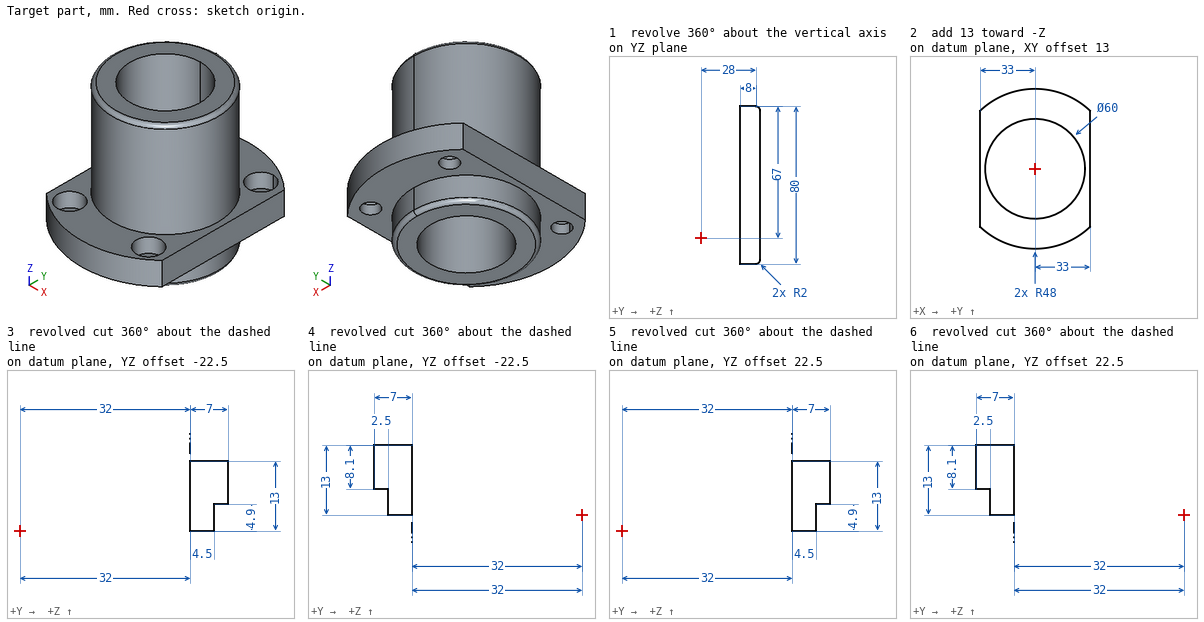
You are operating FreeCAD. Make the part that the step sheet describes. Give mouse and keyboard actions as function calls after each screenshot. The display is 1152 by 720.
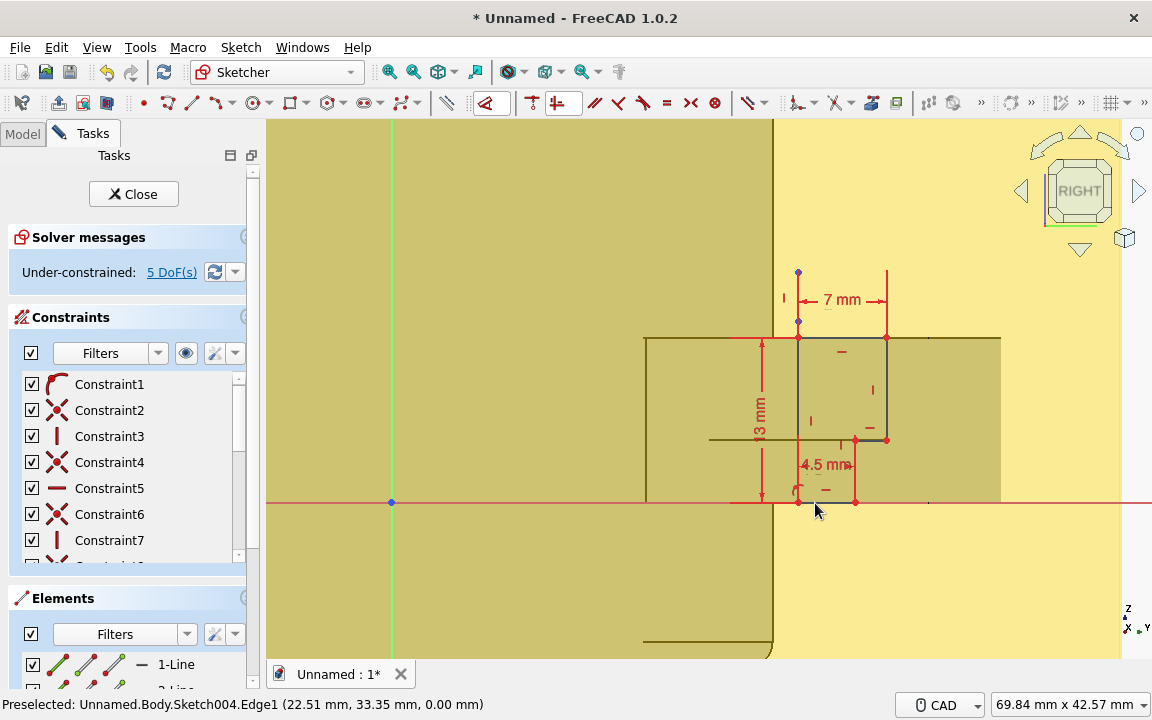
click(855, 484)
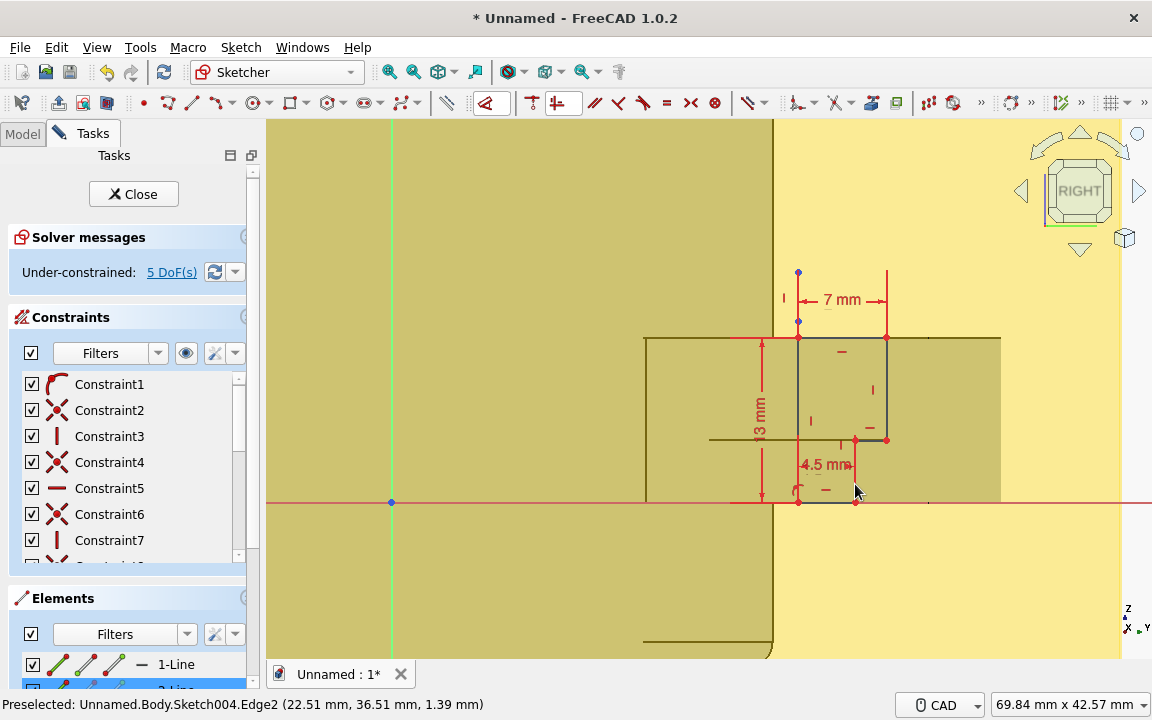
key(i)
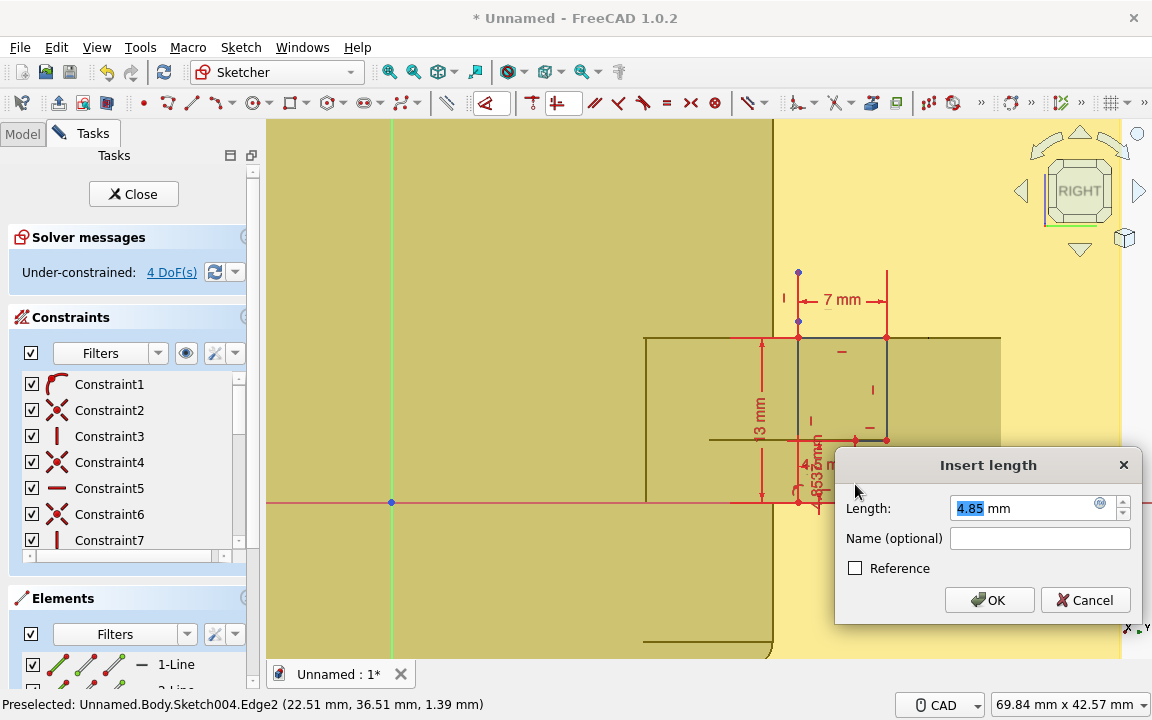
text(4.9)
key(Return)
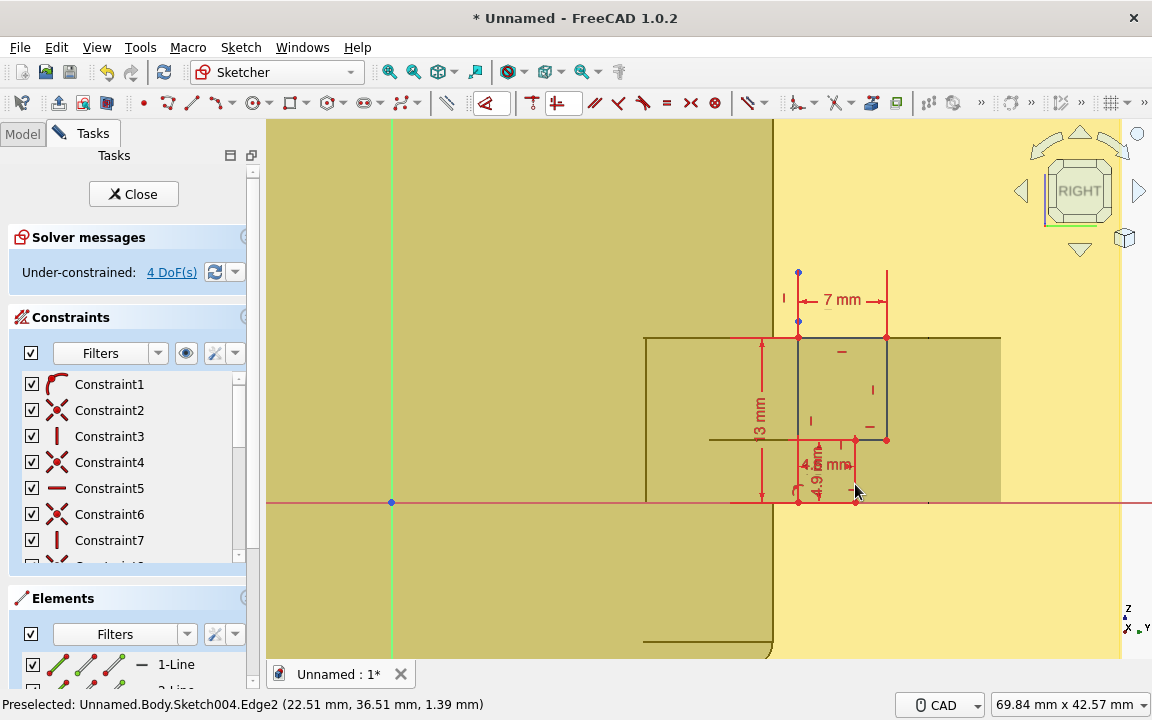
click(798, 503)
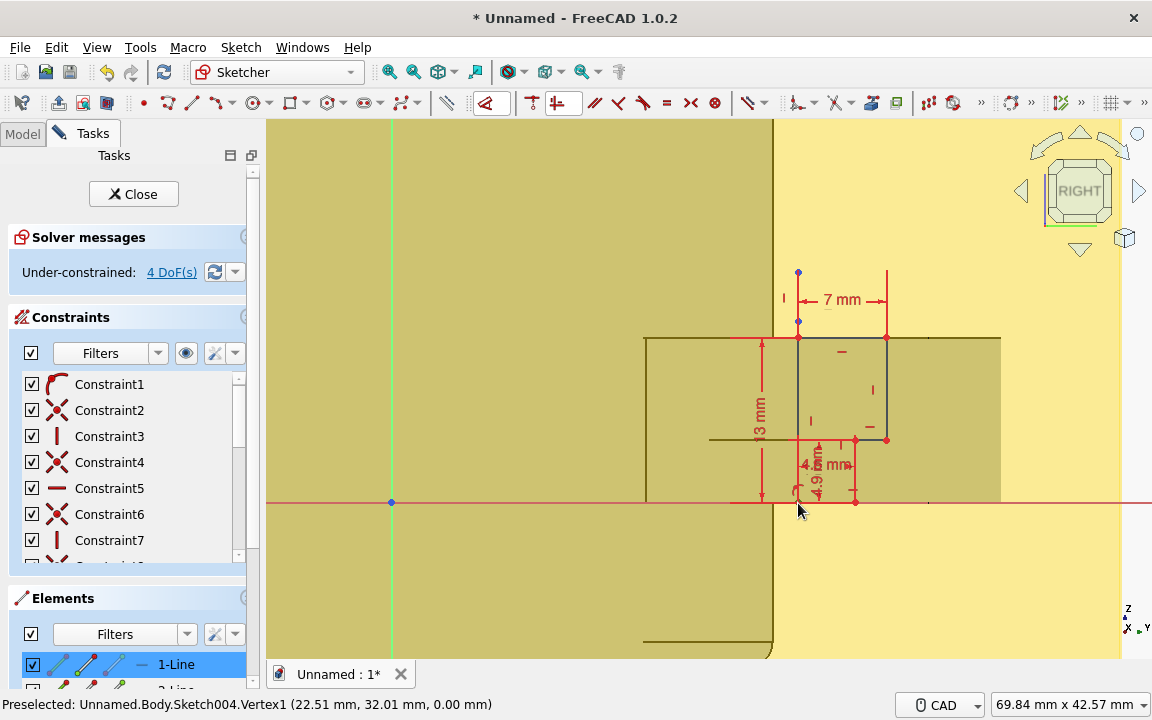
key(l)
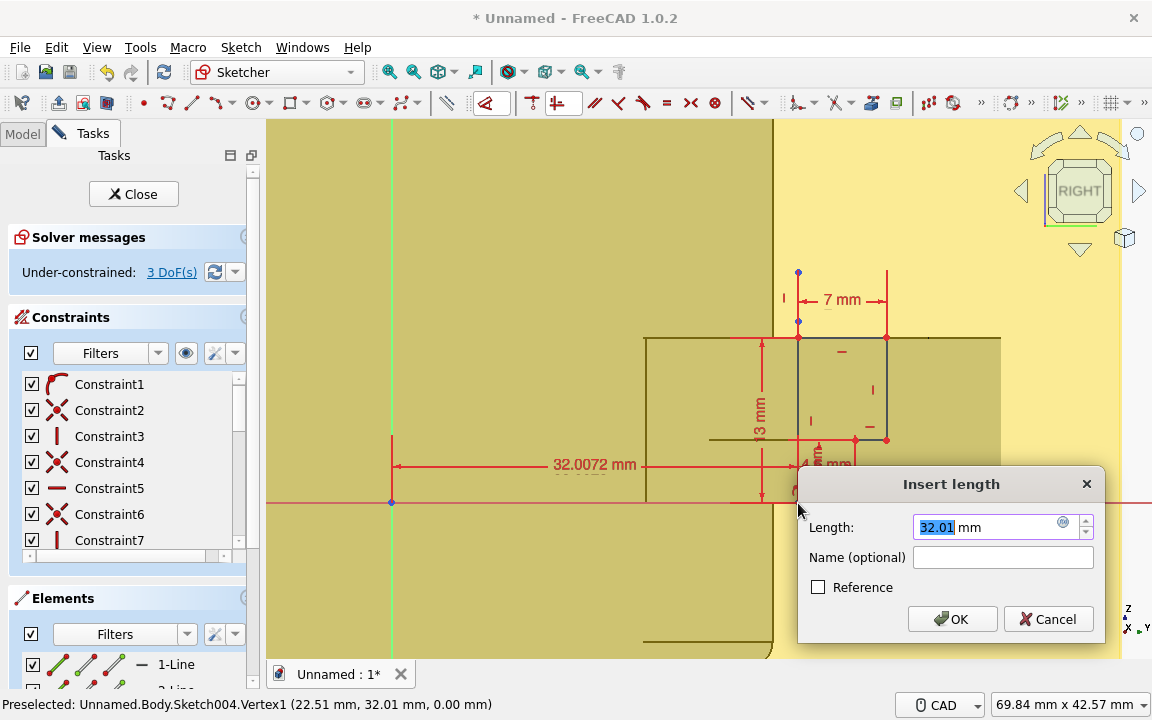
text(32)
key(Return)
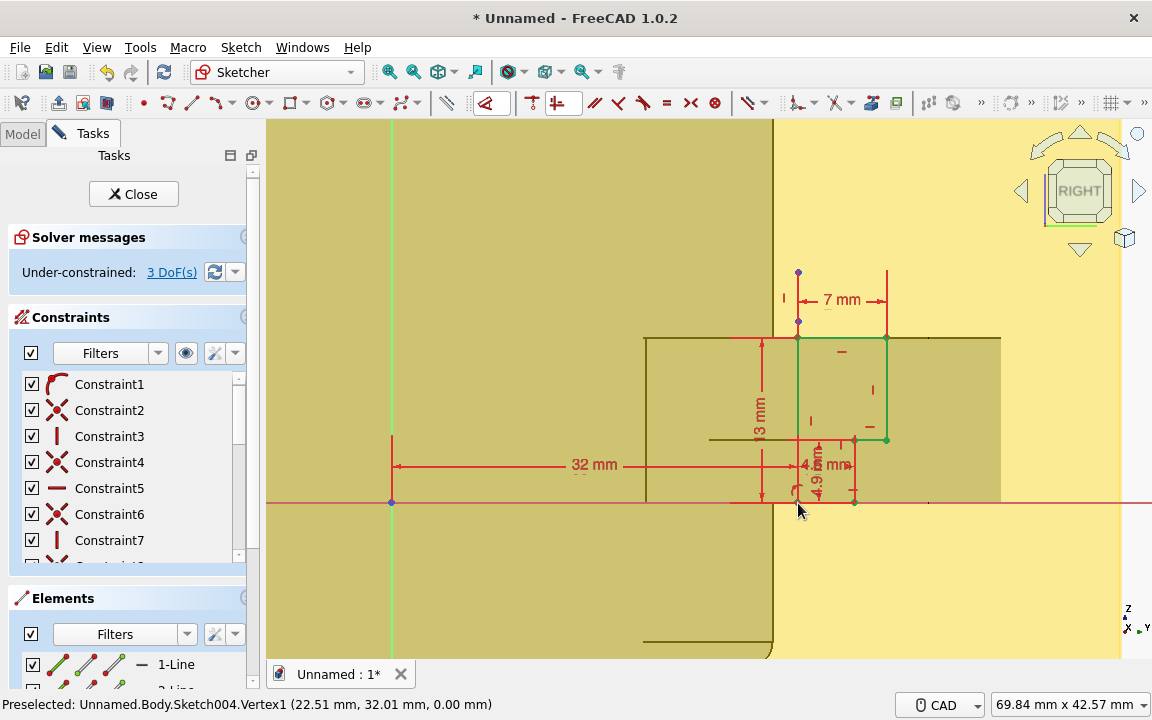
click(798, 322)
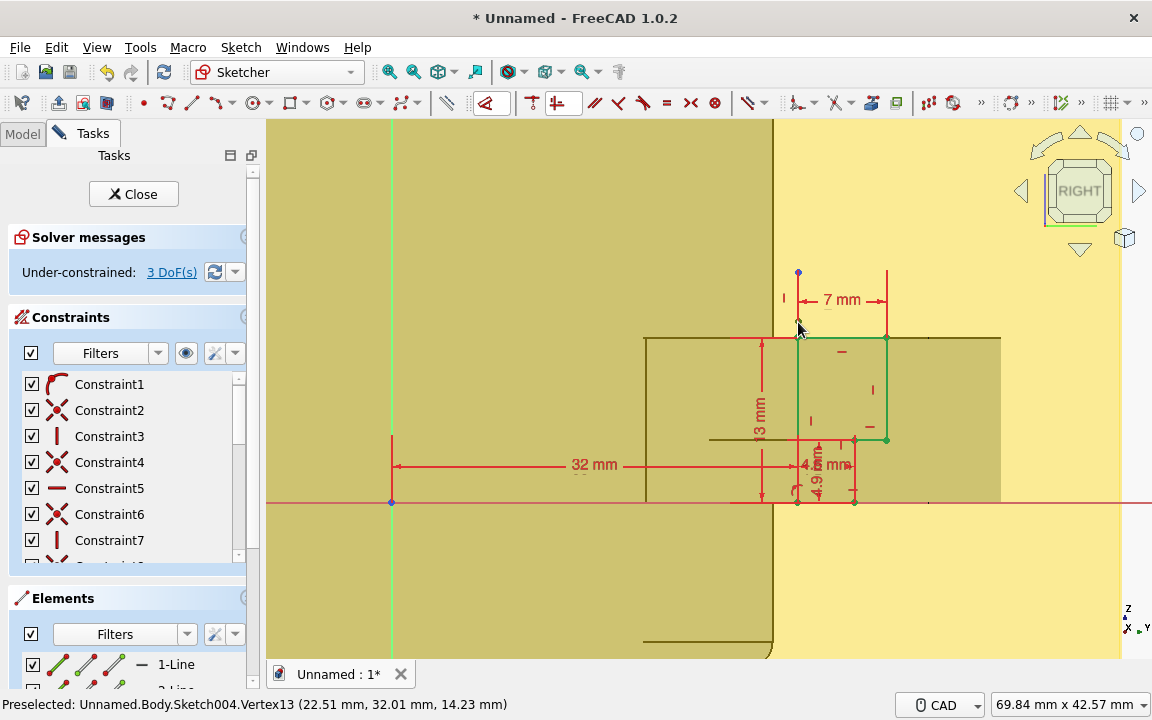
click(504, 104)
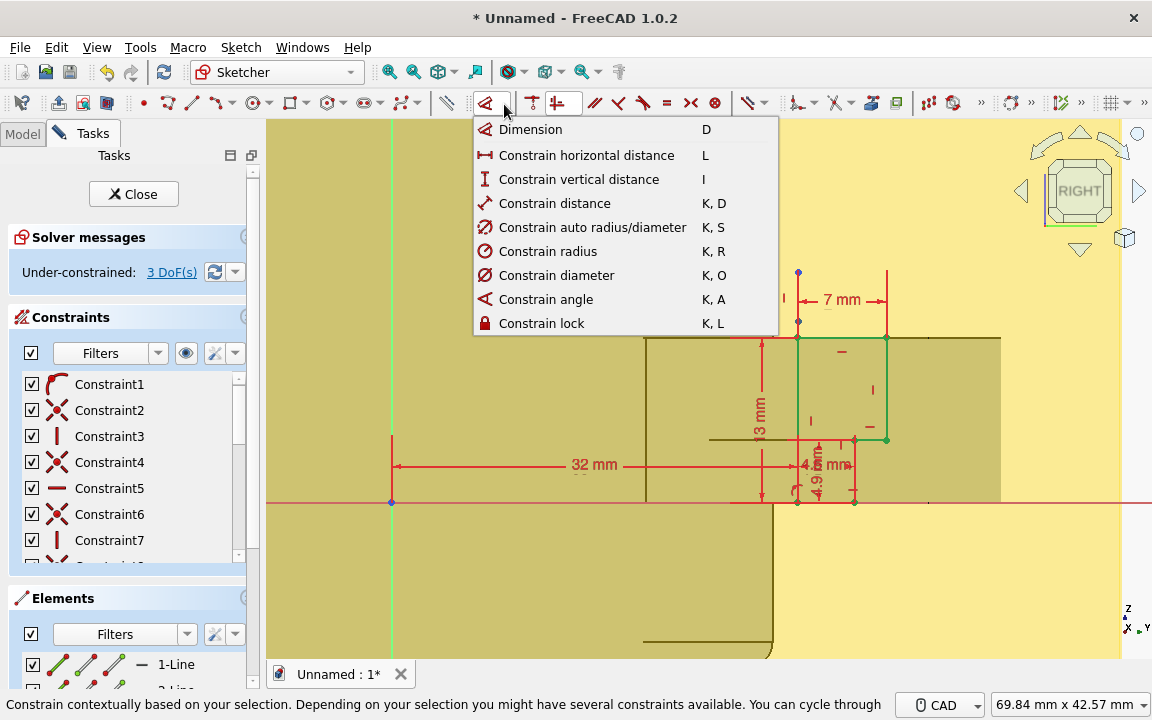
click(626, 155)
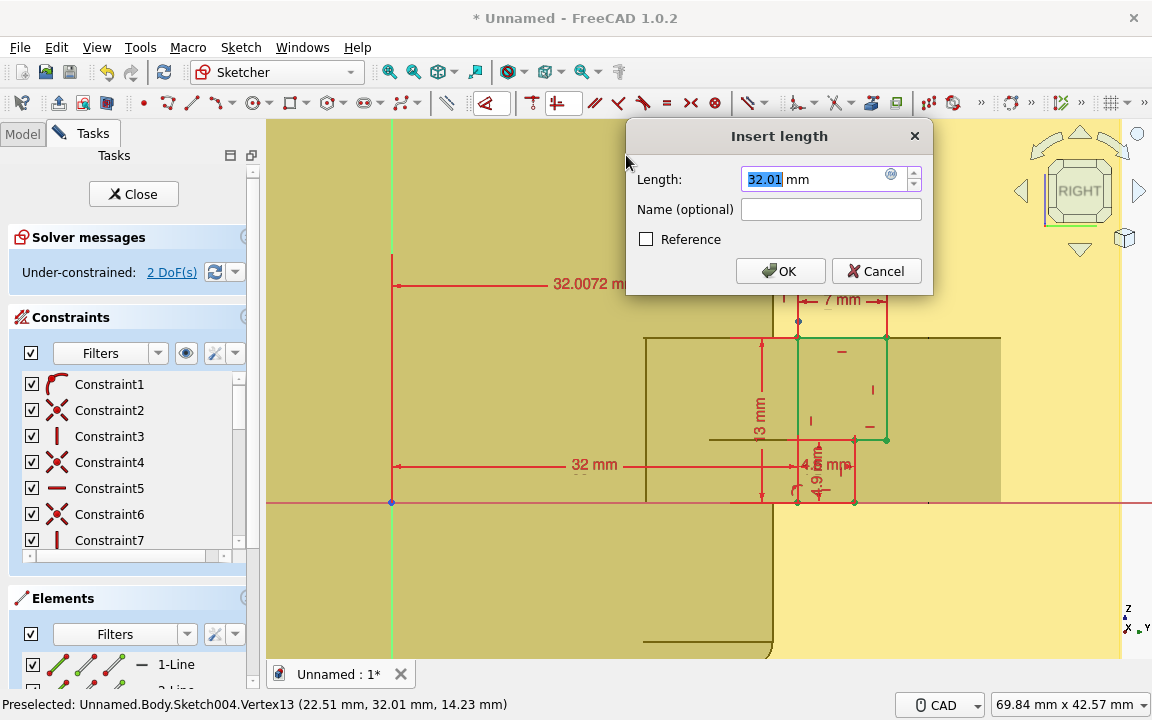
text(32)
key(Return)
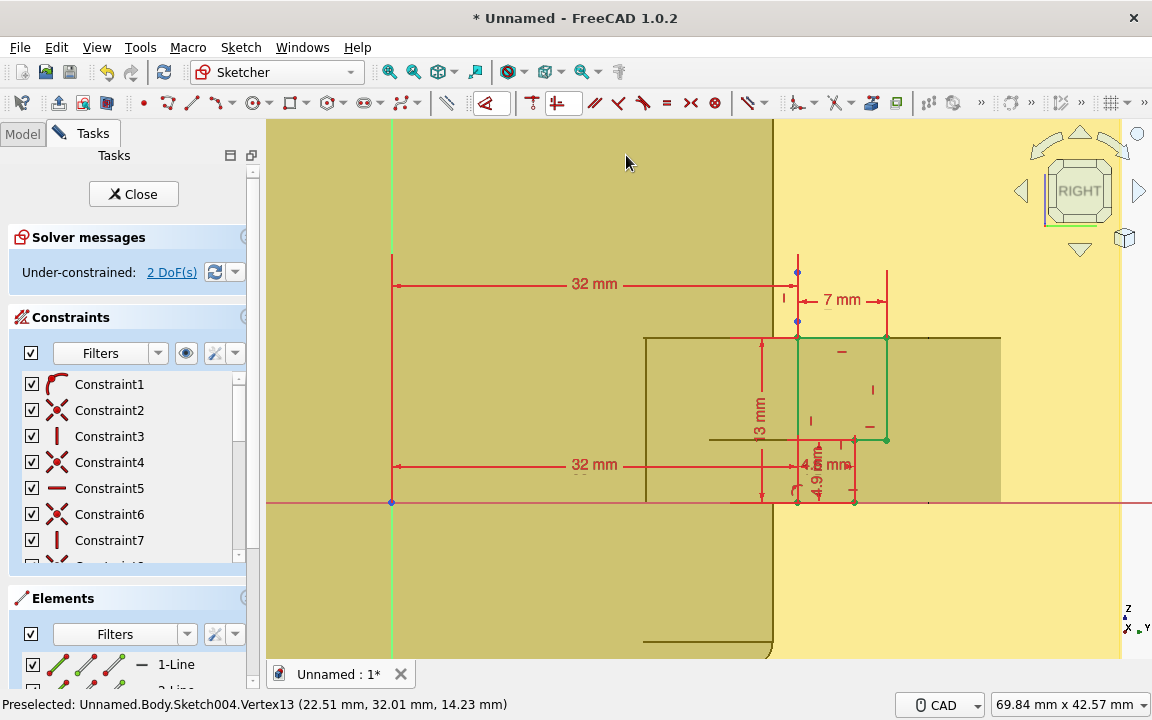
click(134, 194)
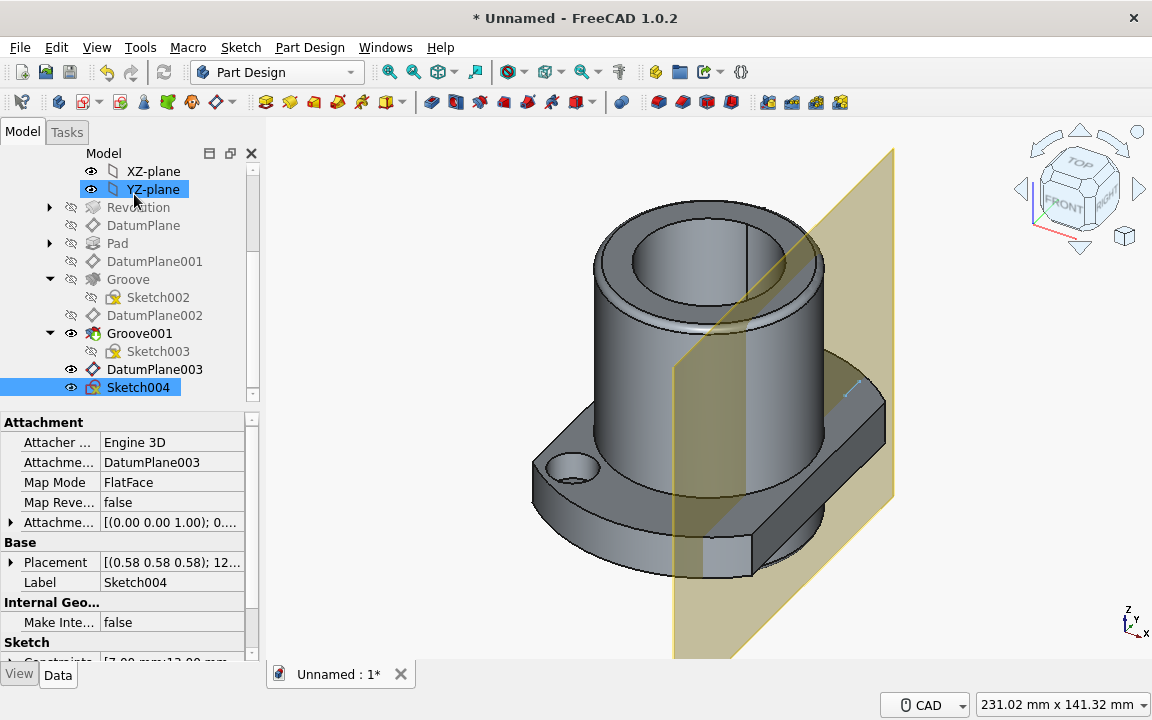
click(480, 102)